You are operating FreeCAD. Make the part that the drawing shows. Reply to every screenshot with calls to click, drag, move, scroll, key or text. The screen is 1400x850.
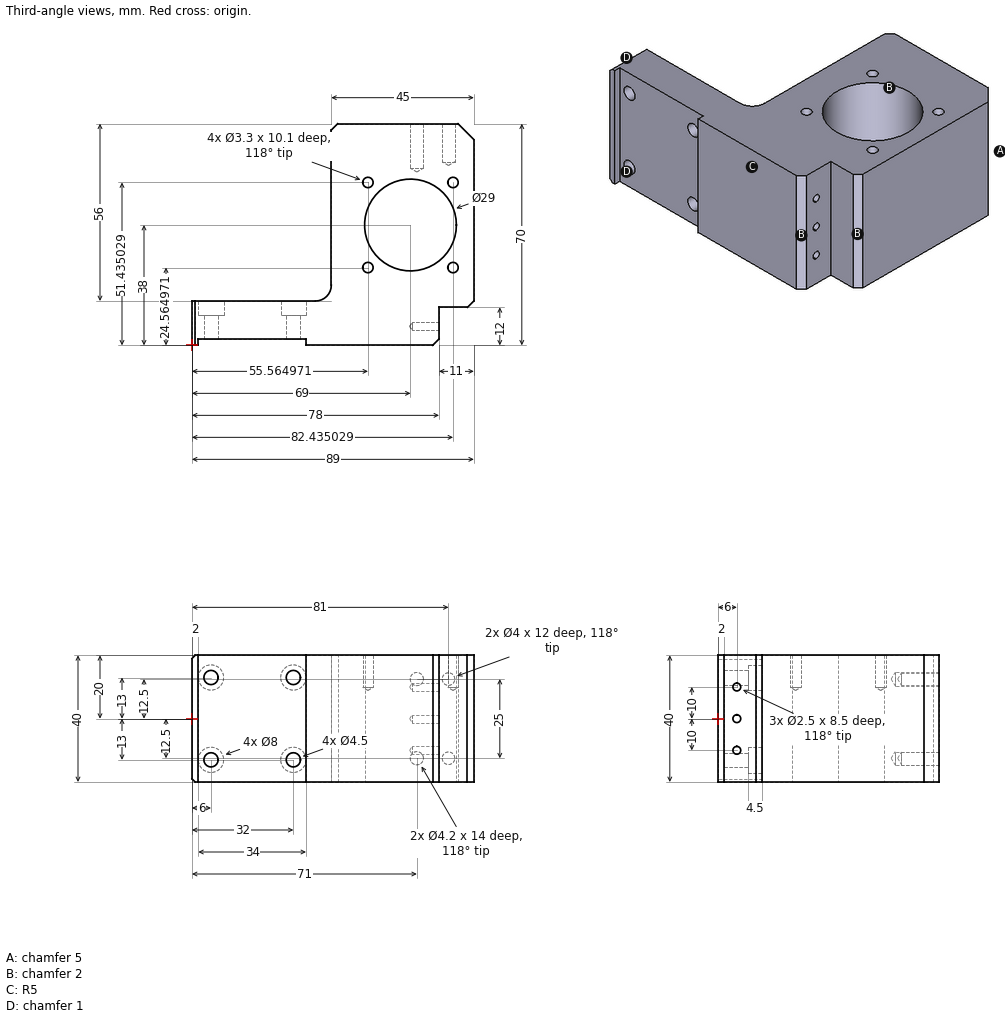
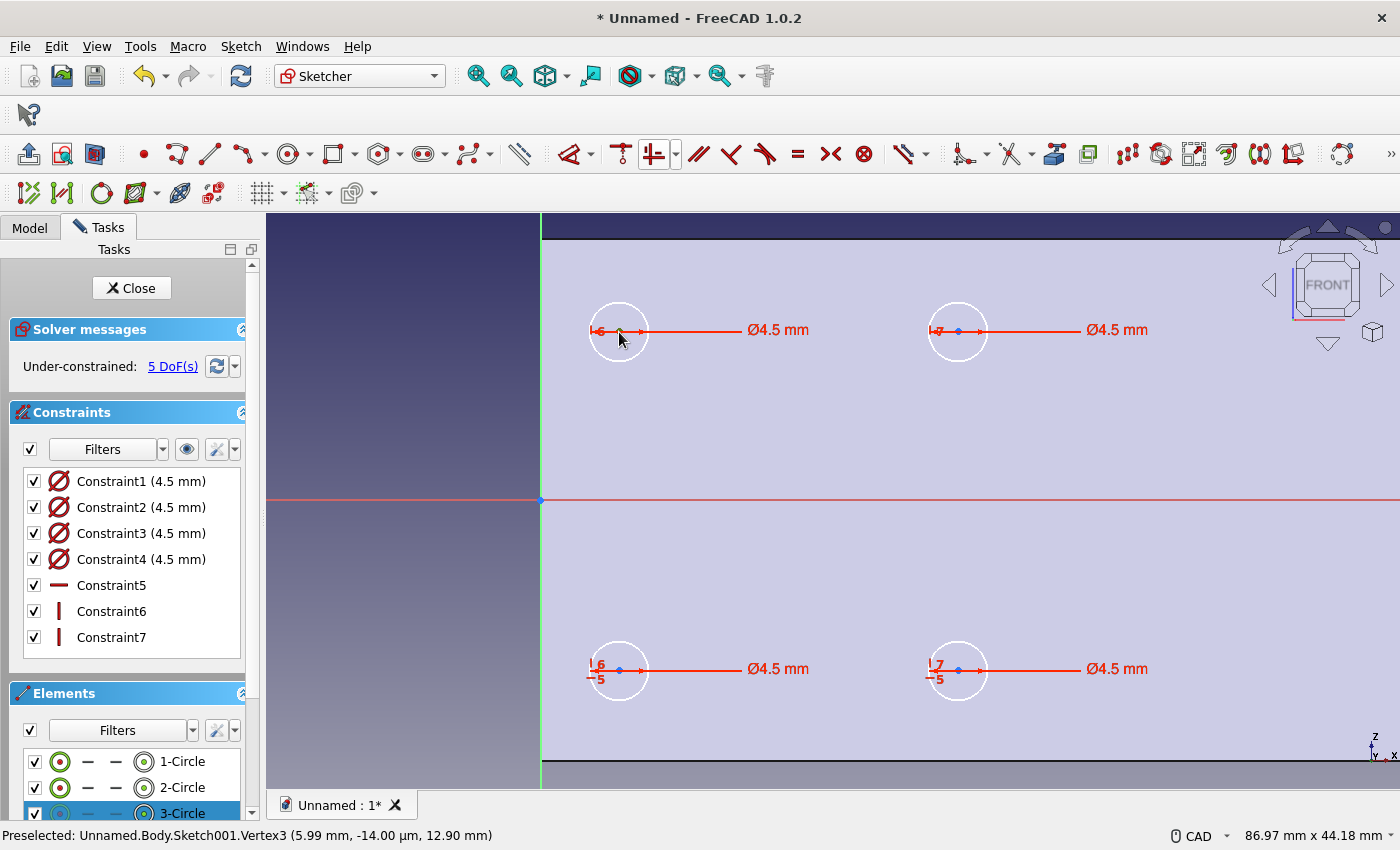
click(958, 332)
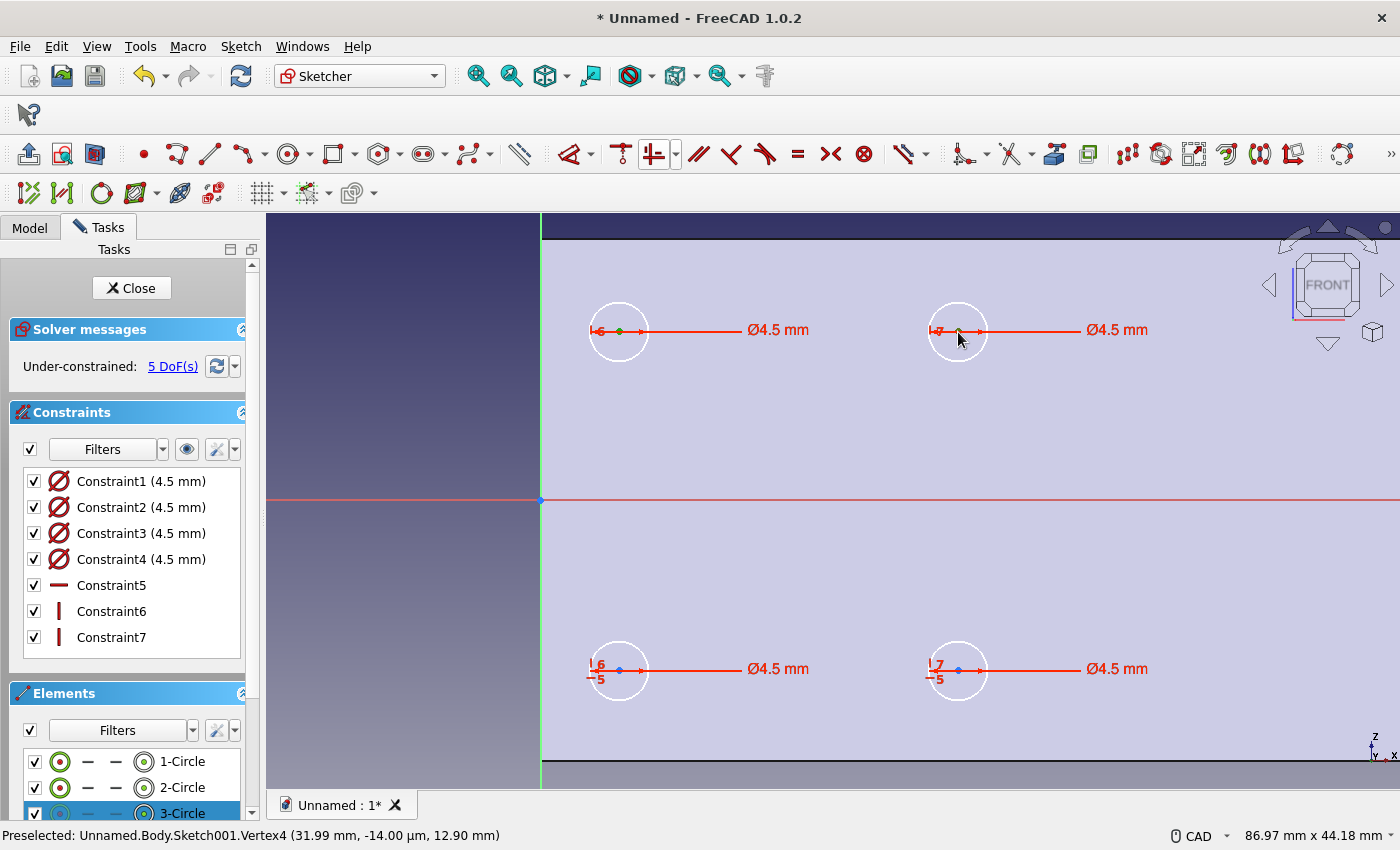
click(676, 154)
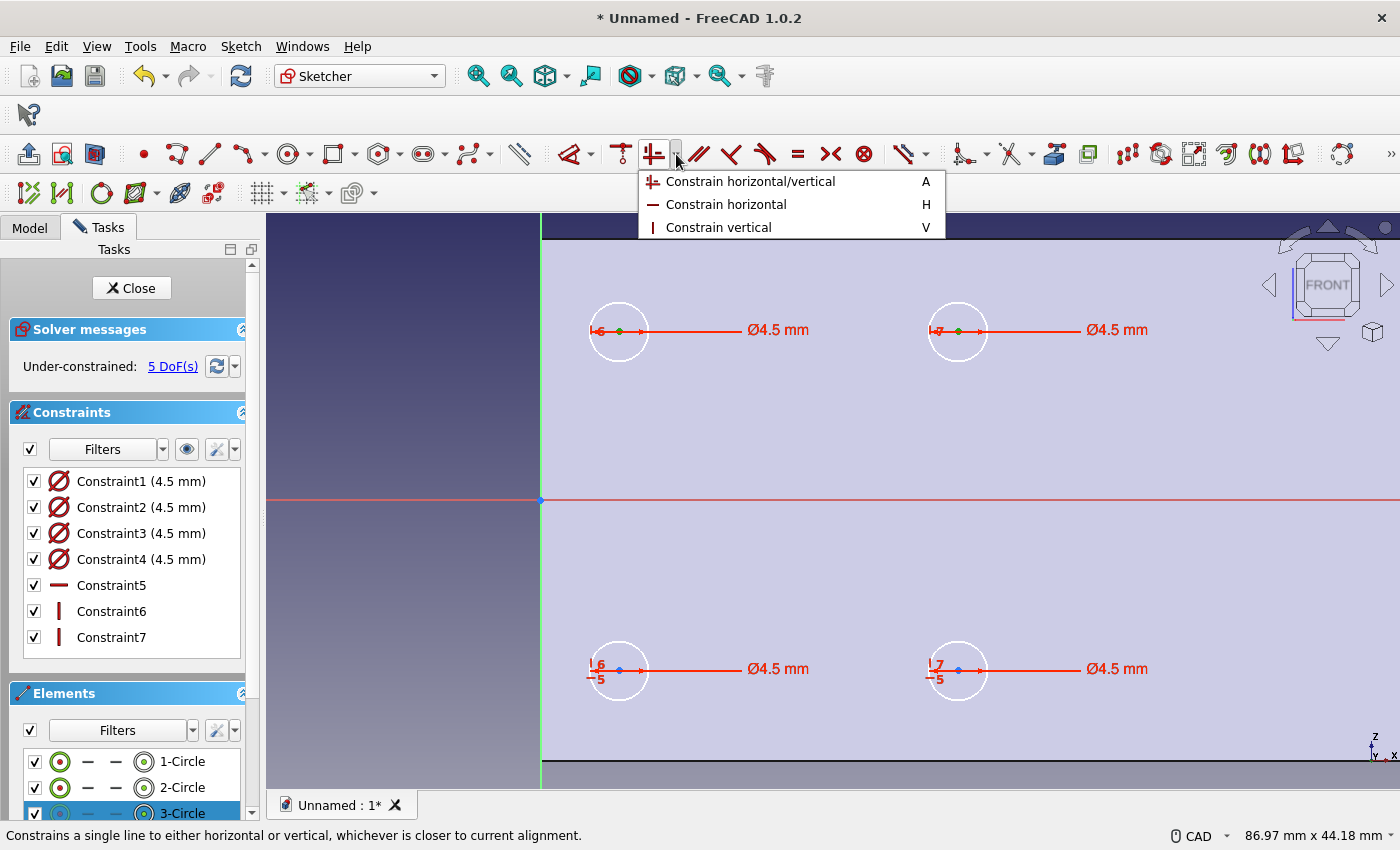
click(792, 204)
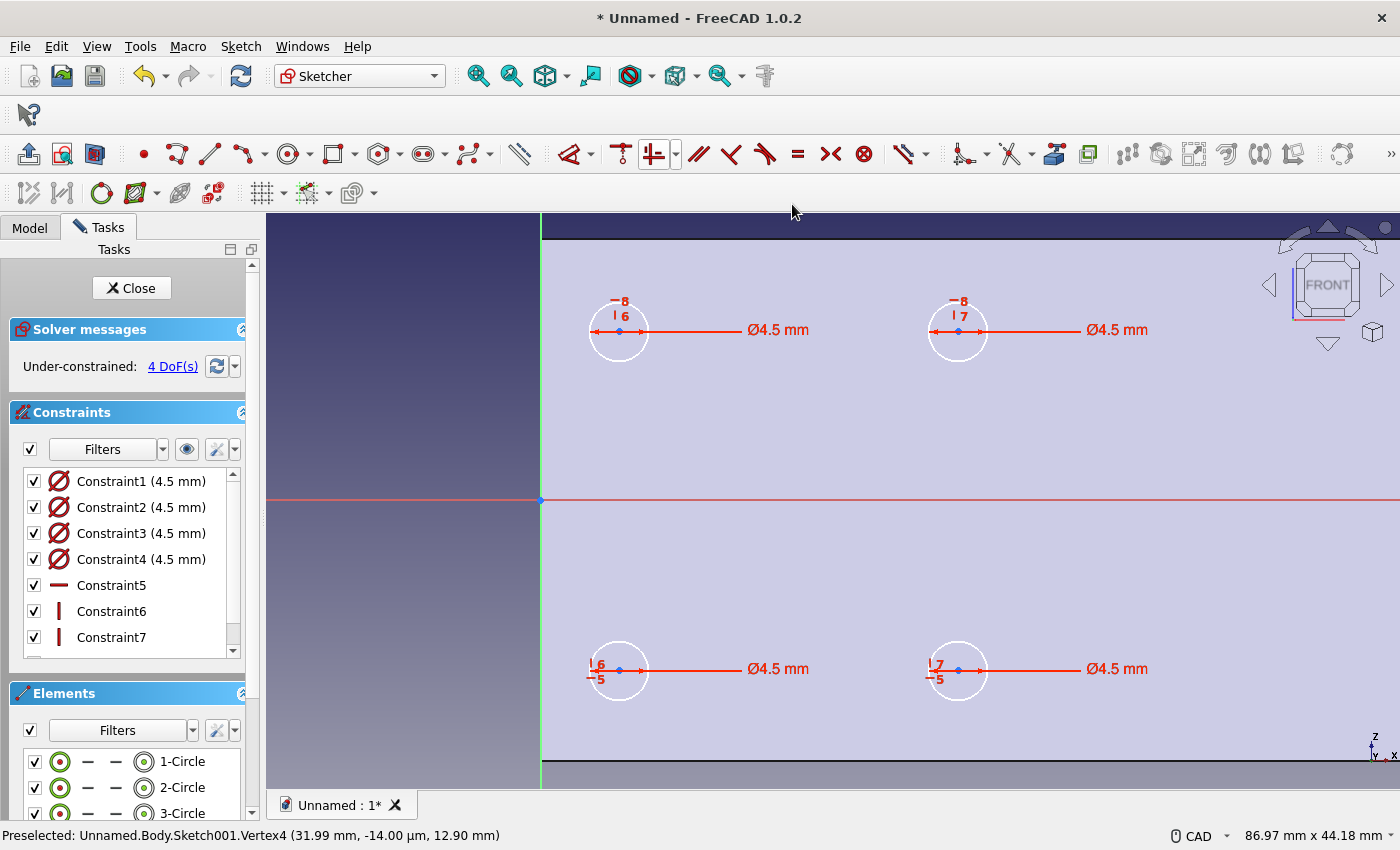
key(d)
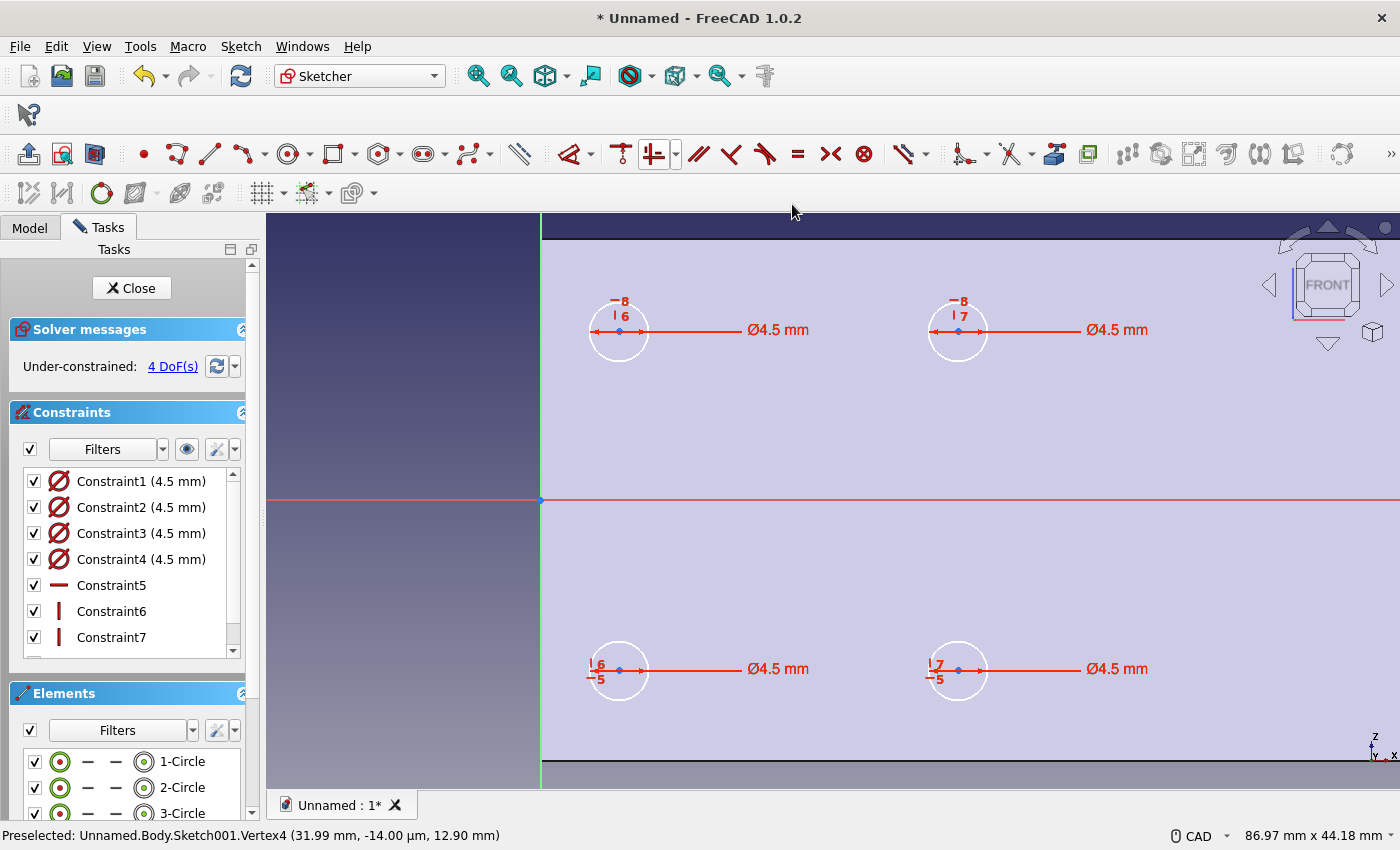
click(619, 671)
click(580, 705)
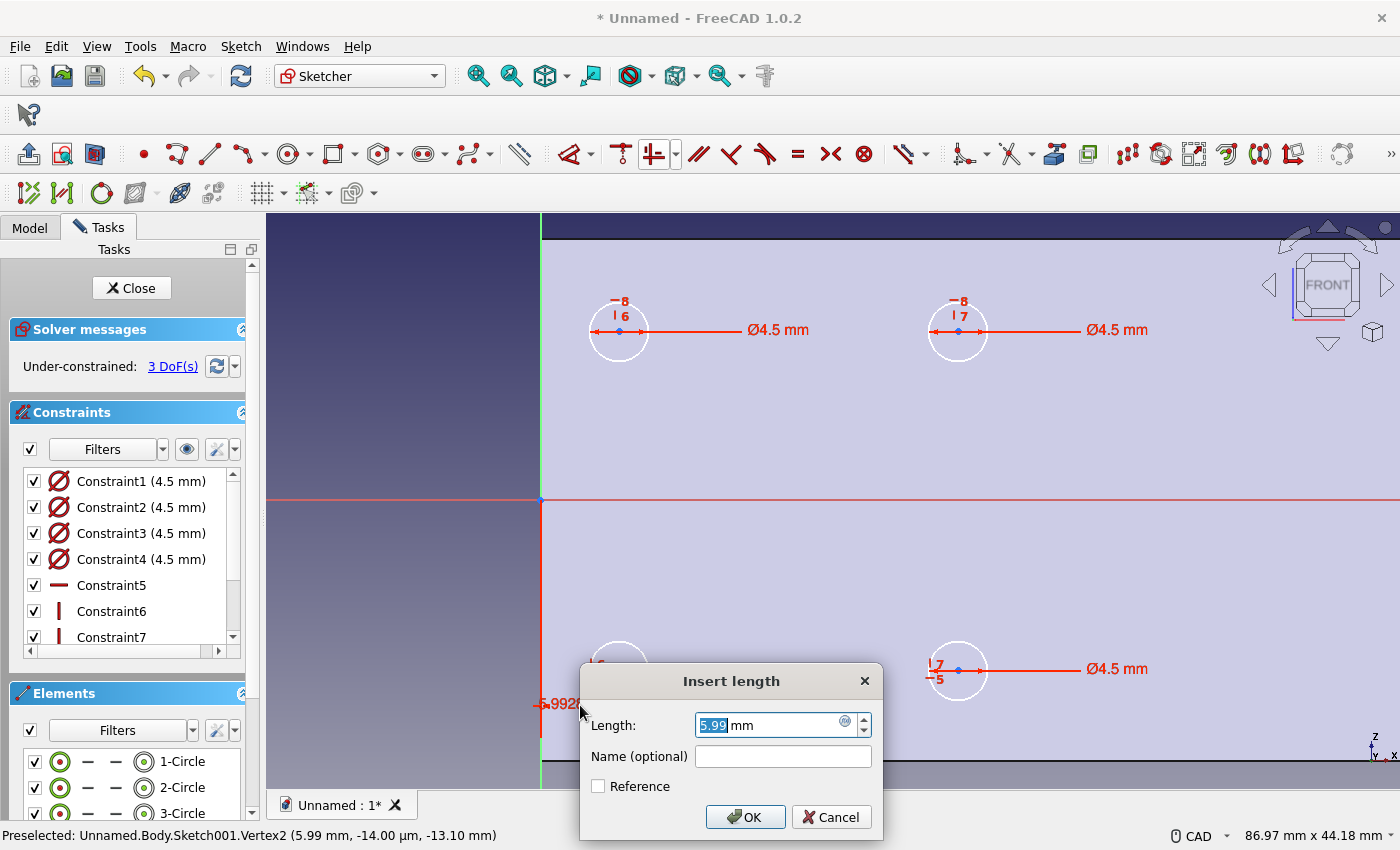
text(6)
key(Return)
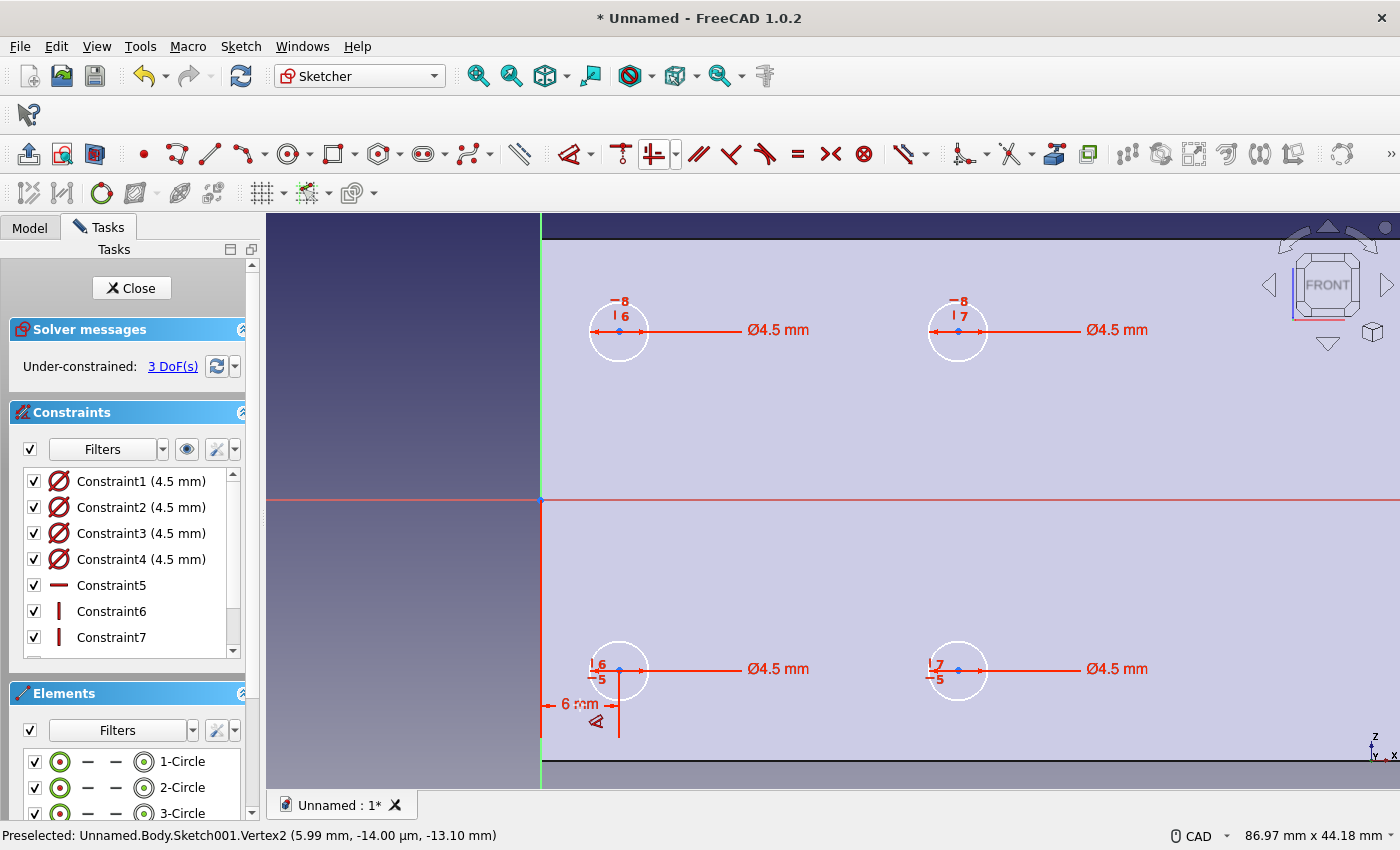
click(958, 671)
click(749, 705)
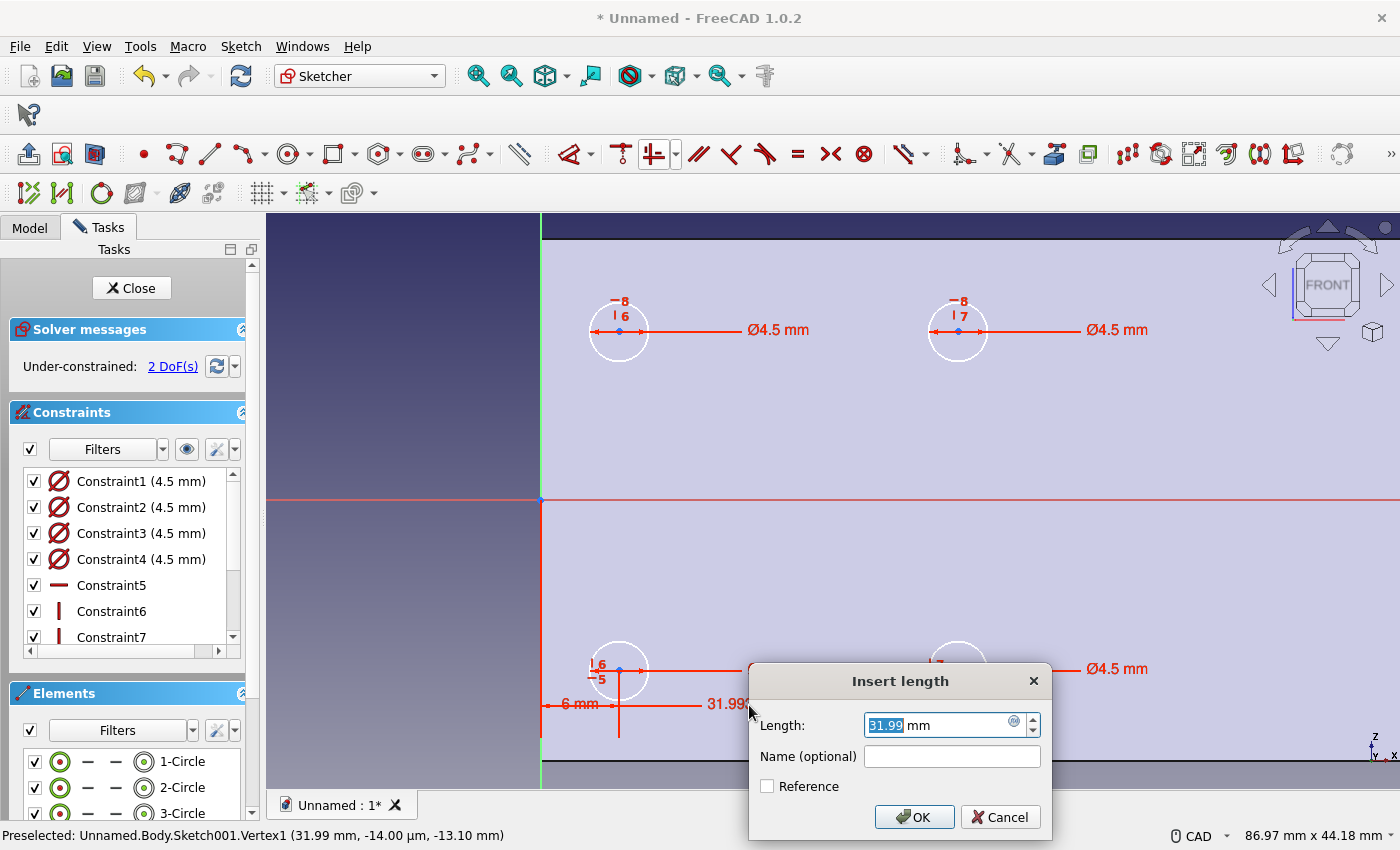
text(32)
key(Return)